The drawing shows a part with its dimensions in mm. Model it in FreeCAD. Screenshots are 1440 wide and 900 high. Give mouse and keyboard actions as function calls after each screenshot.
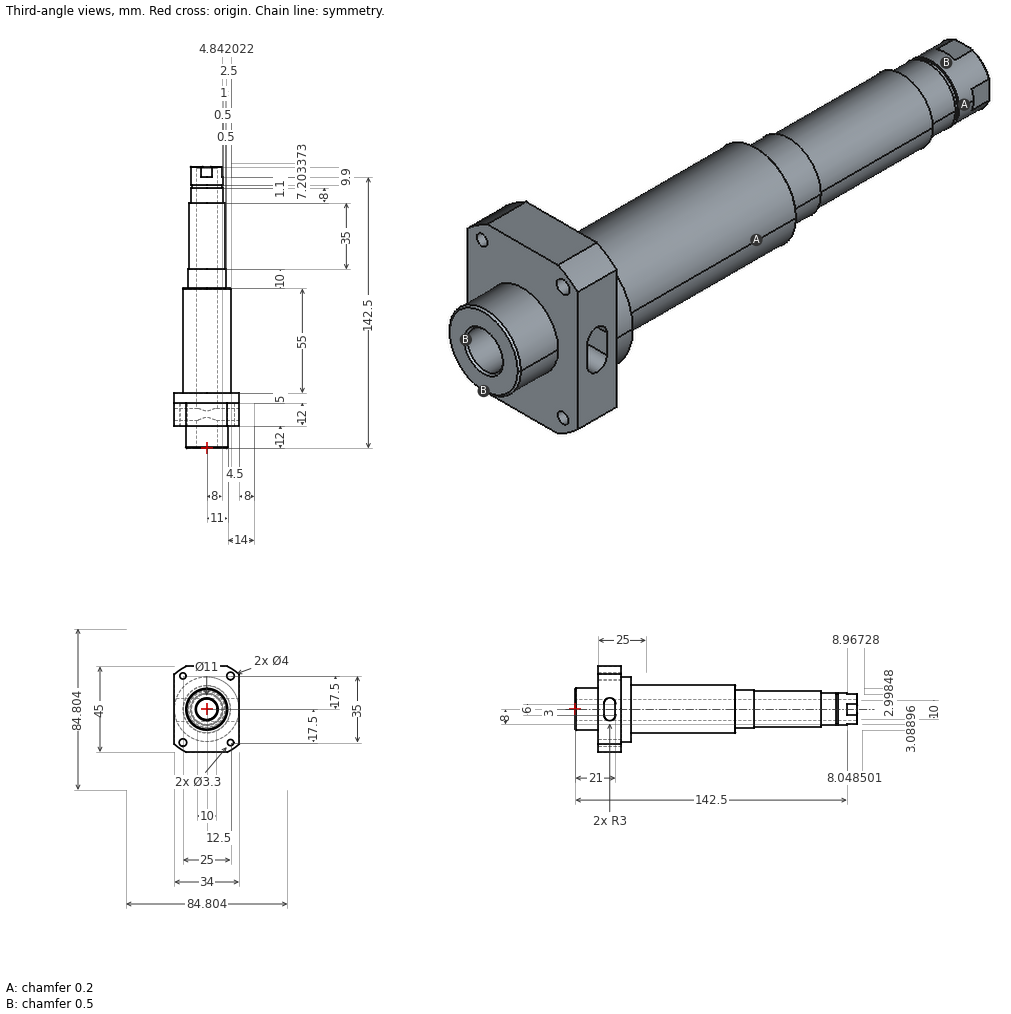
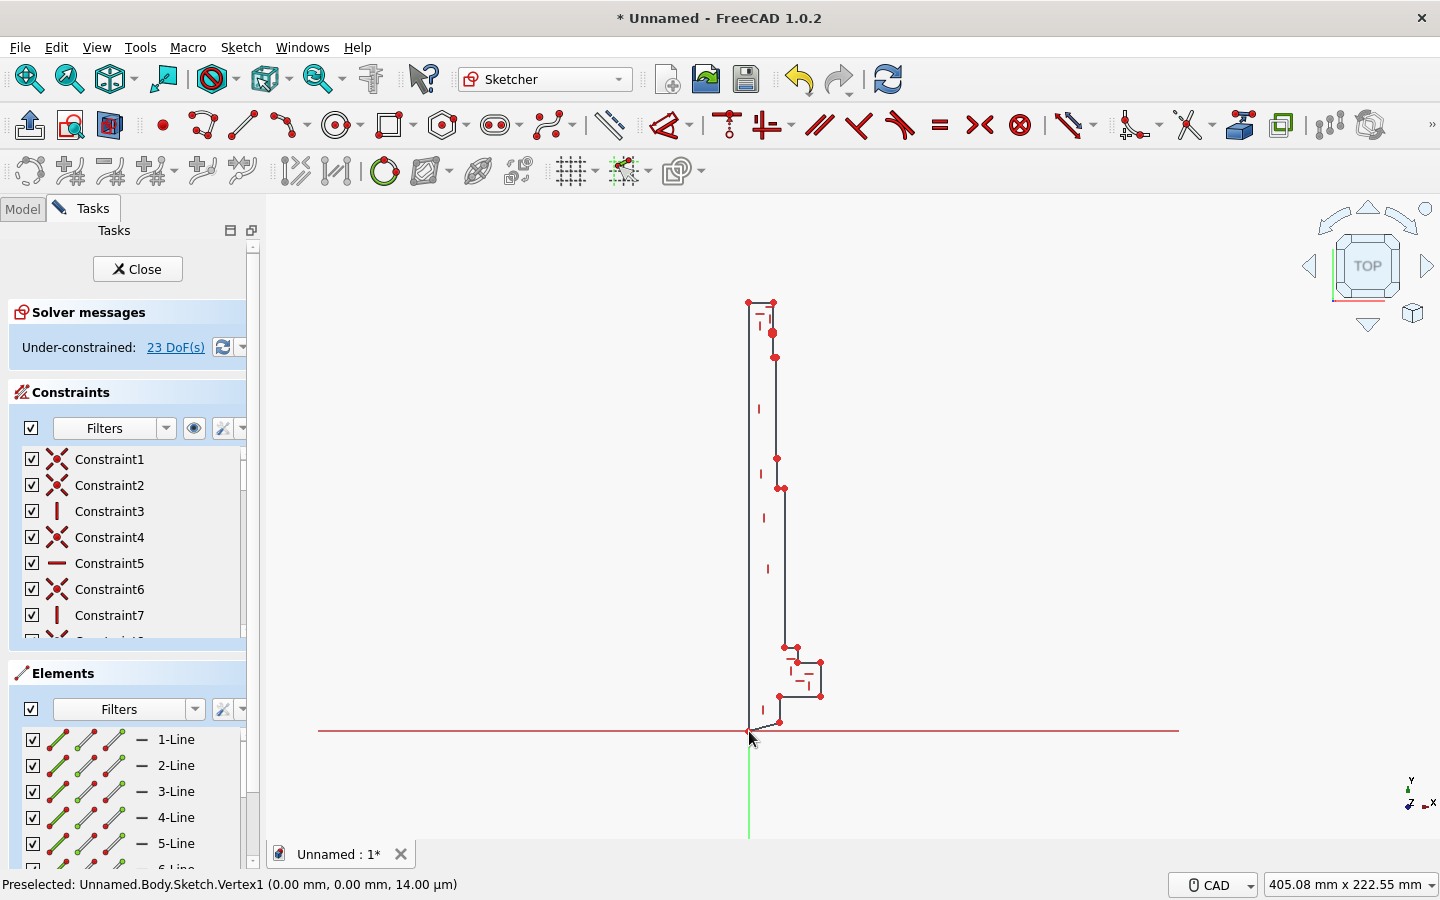
scroll(758, 729, up, 2)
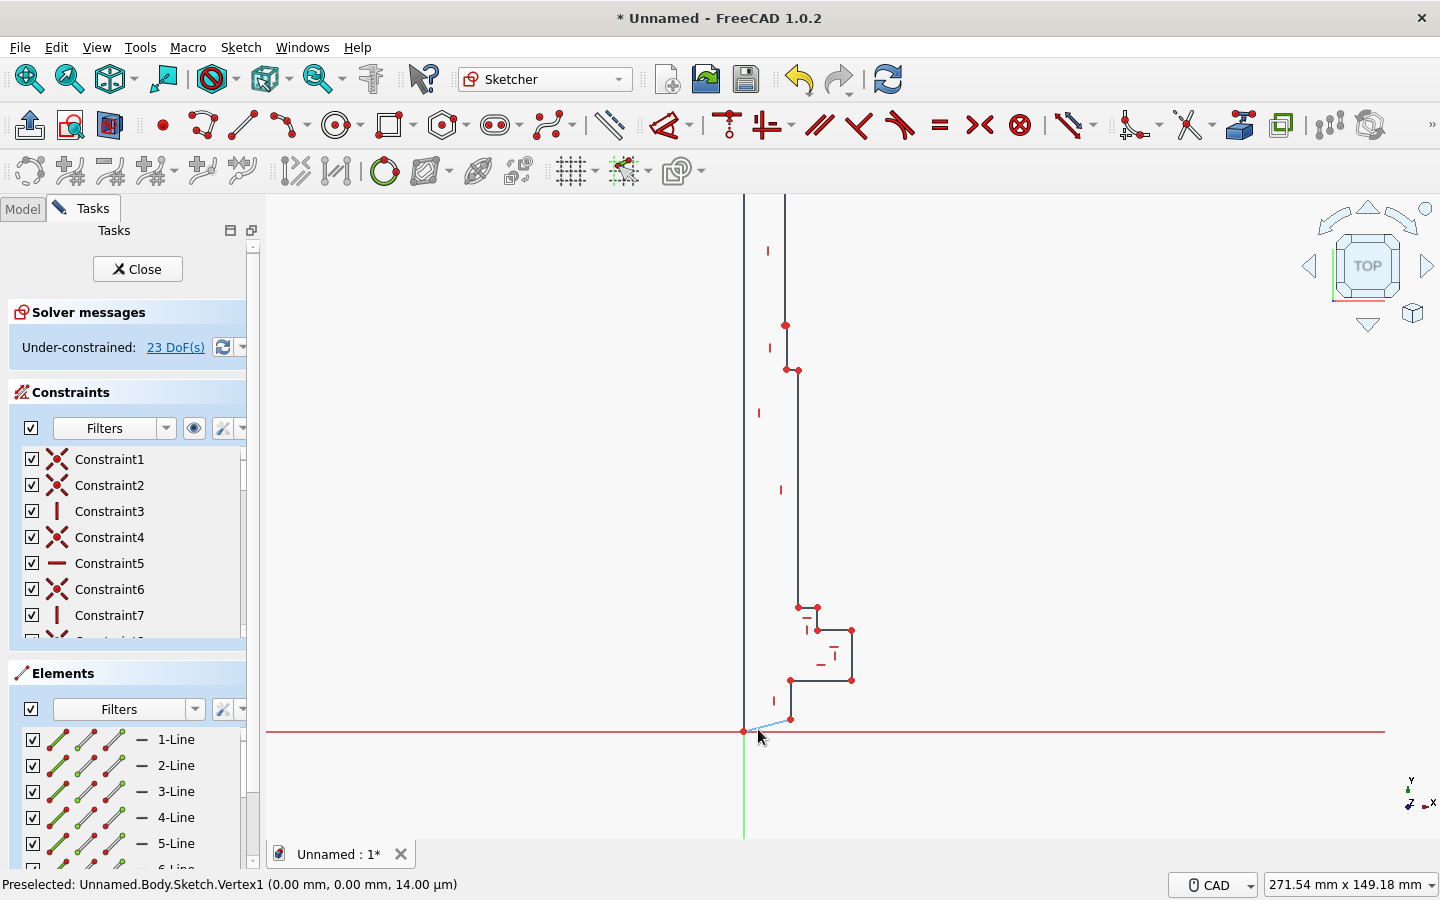
click(758, 728)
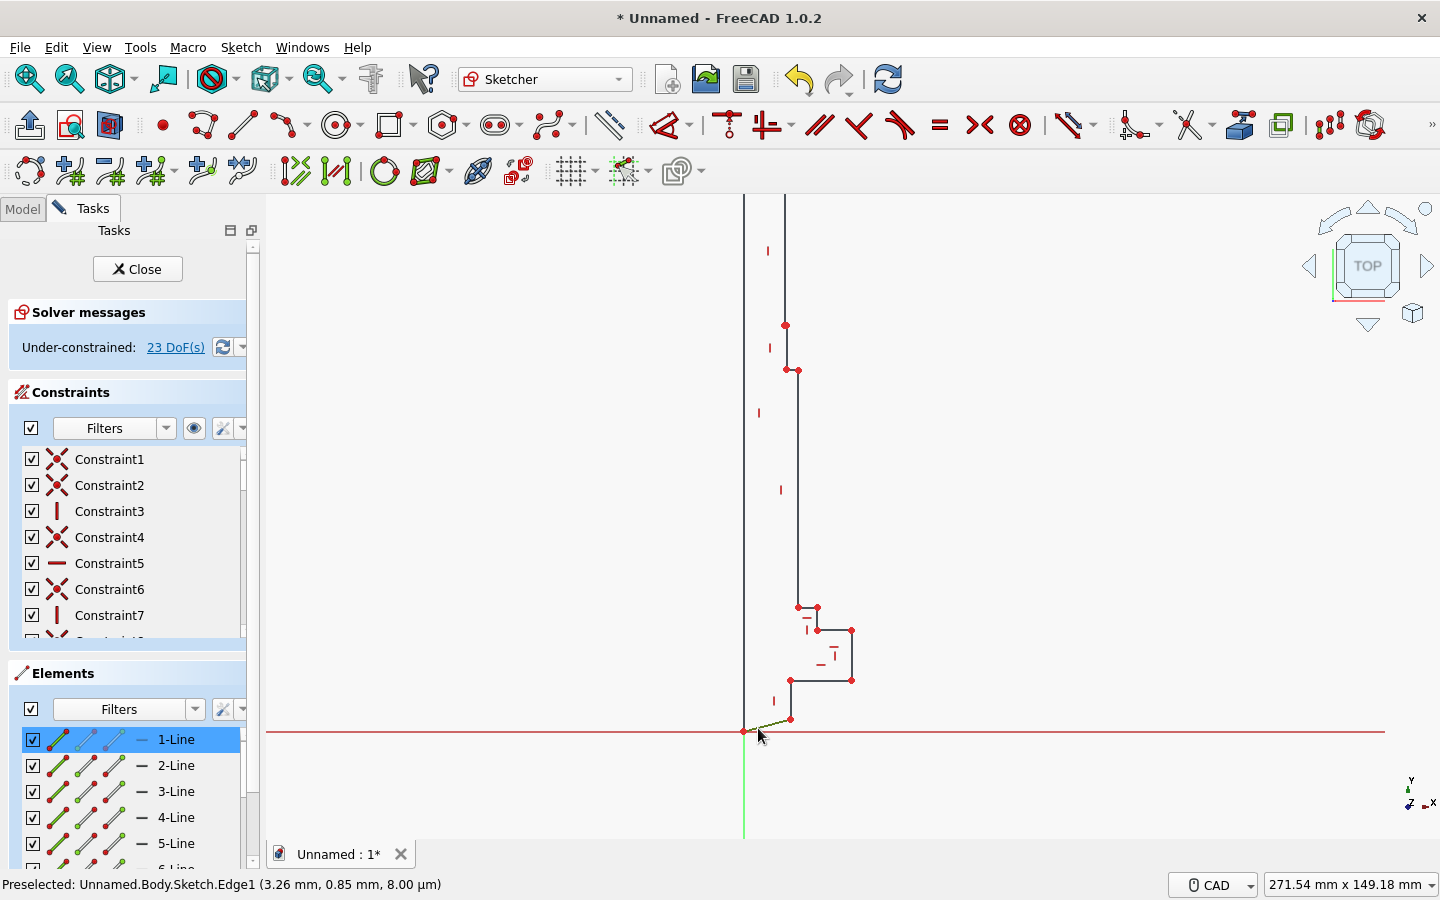
click(794, 126)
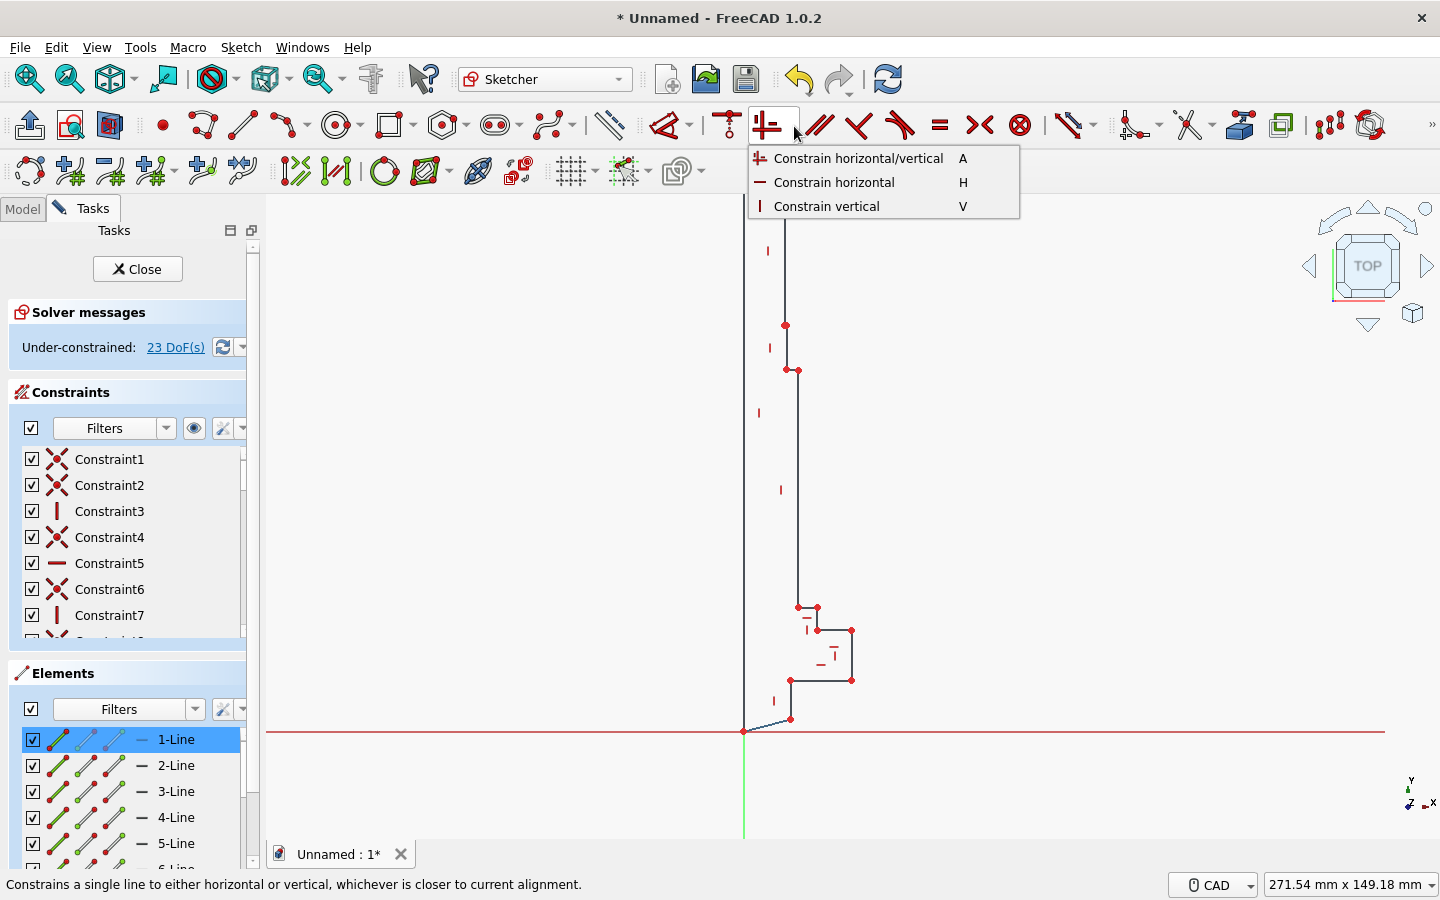
click(884, 182)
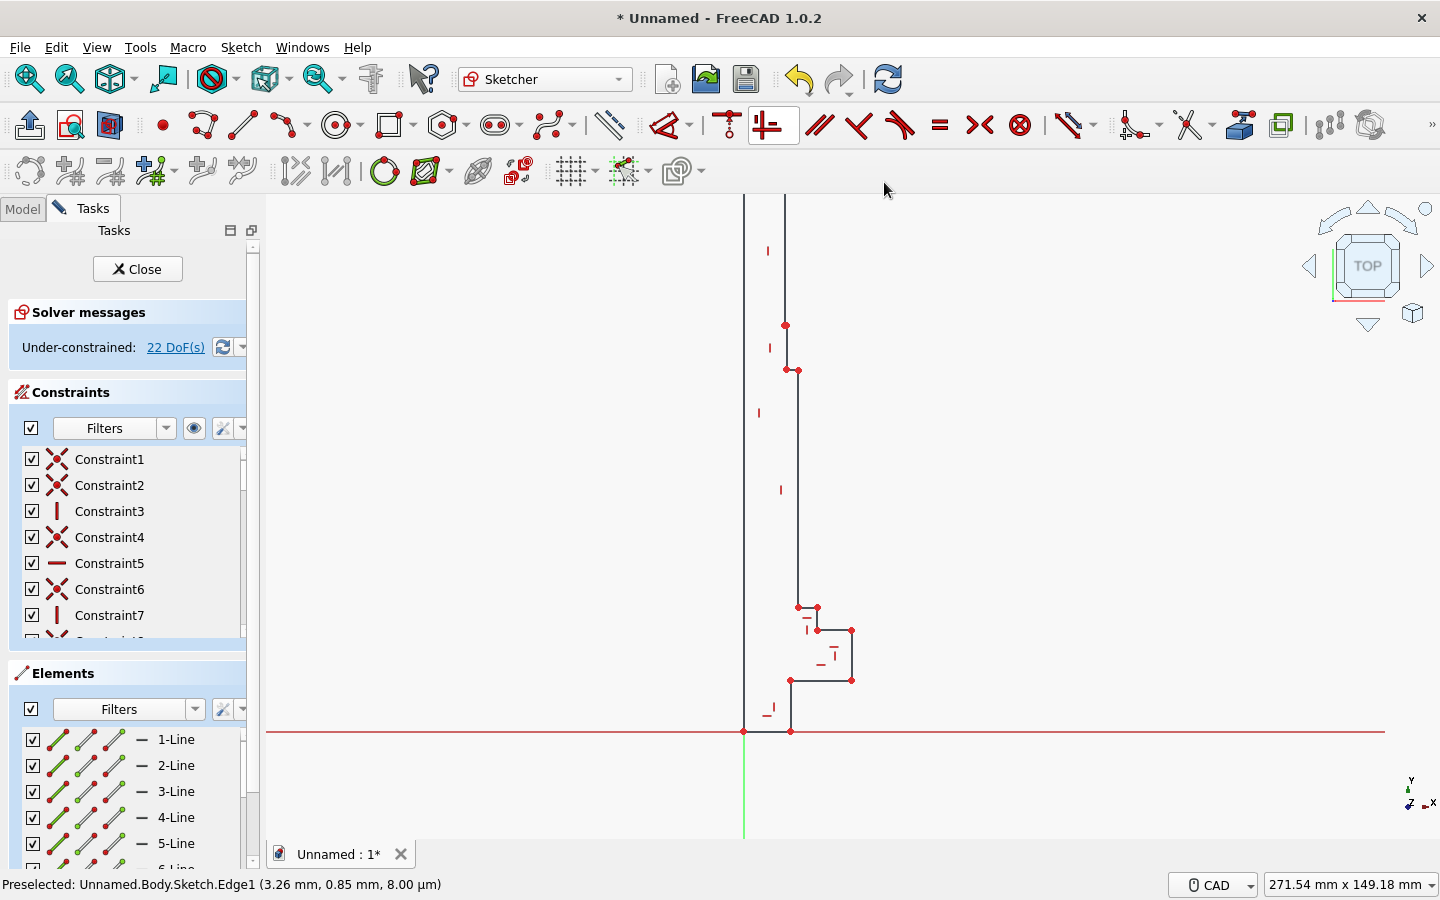
scroll(792, 370, up, 5)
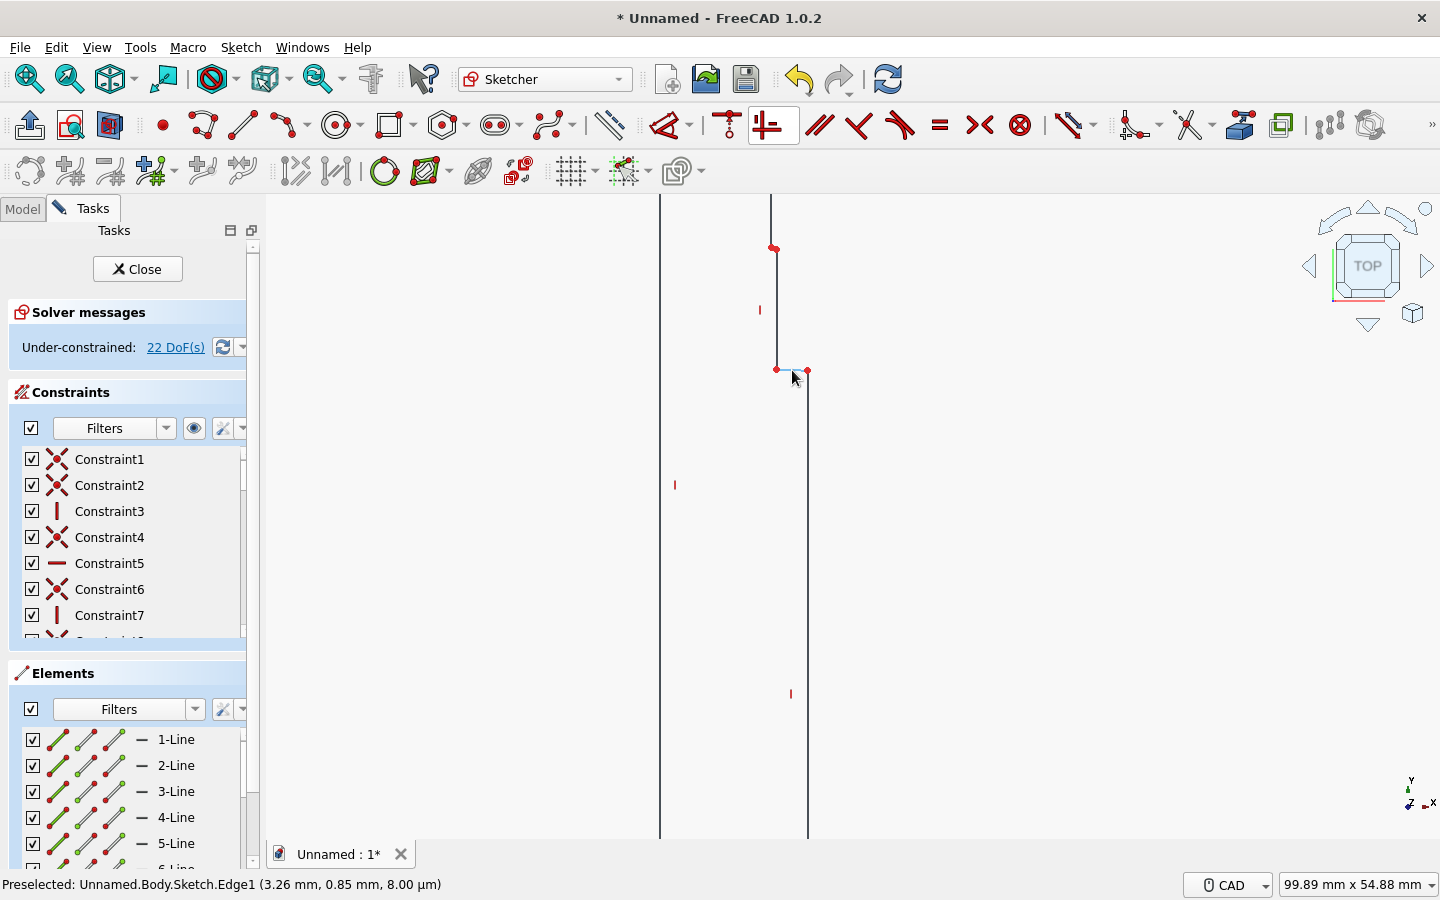
click(792, 370)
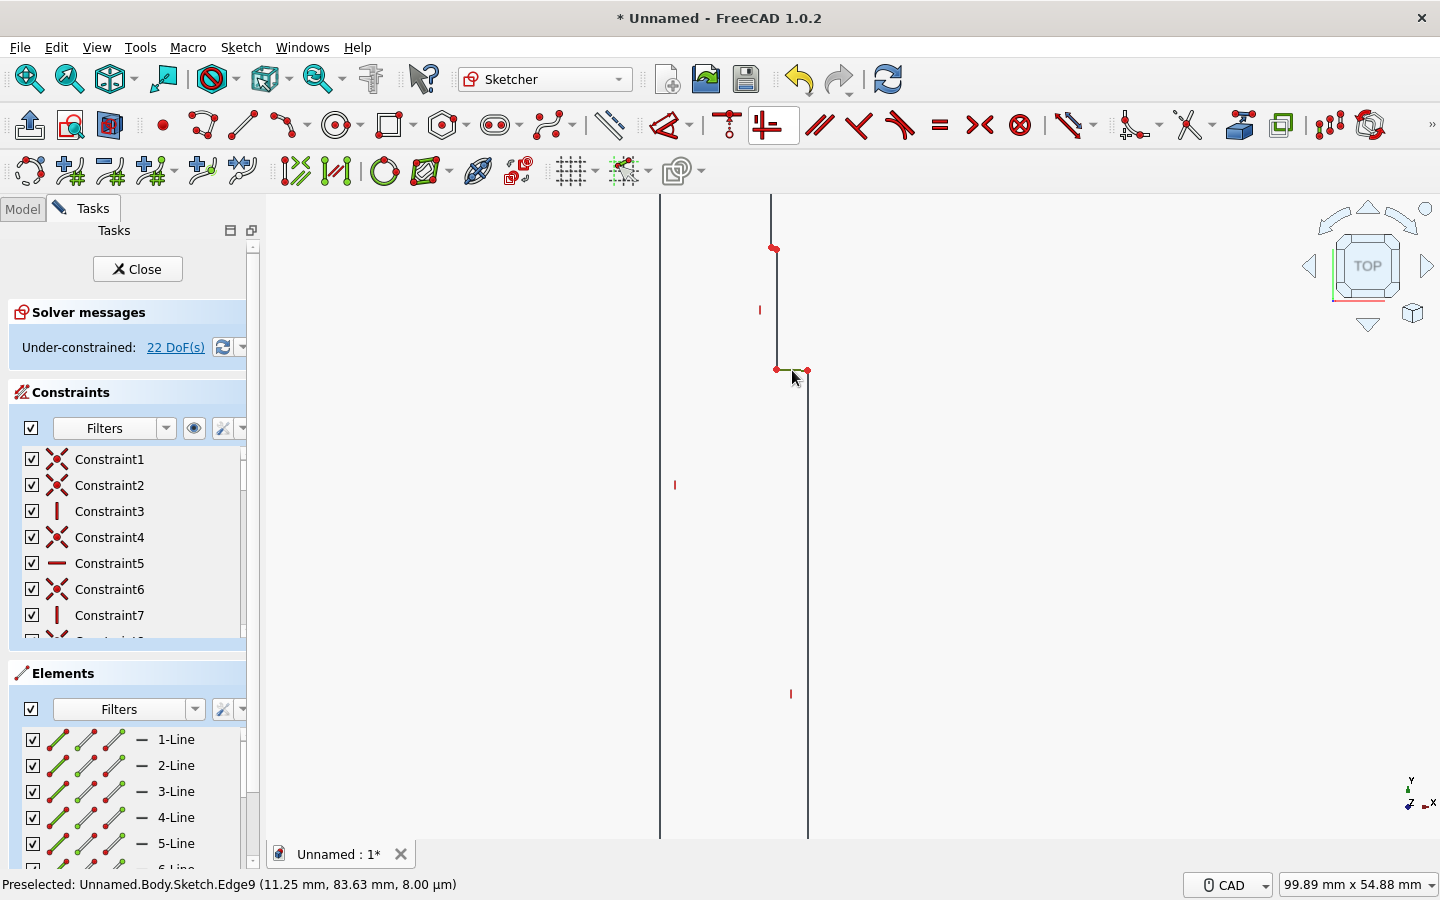
key(h)